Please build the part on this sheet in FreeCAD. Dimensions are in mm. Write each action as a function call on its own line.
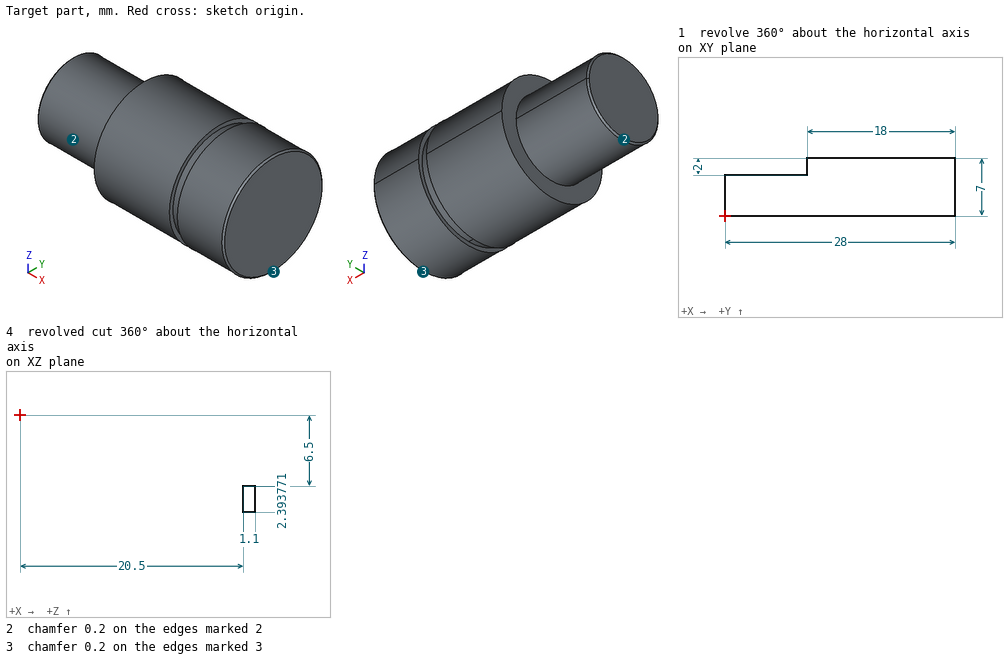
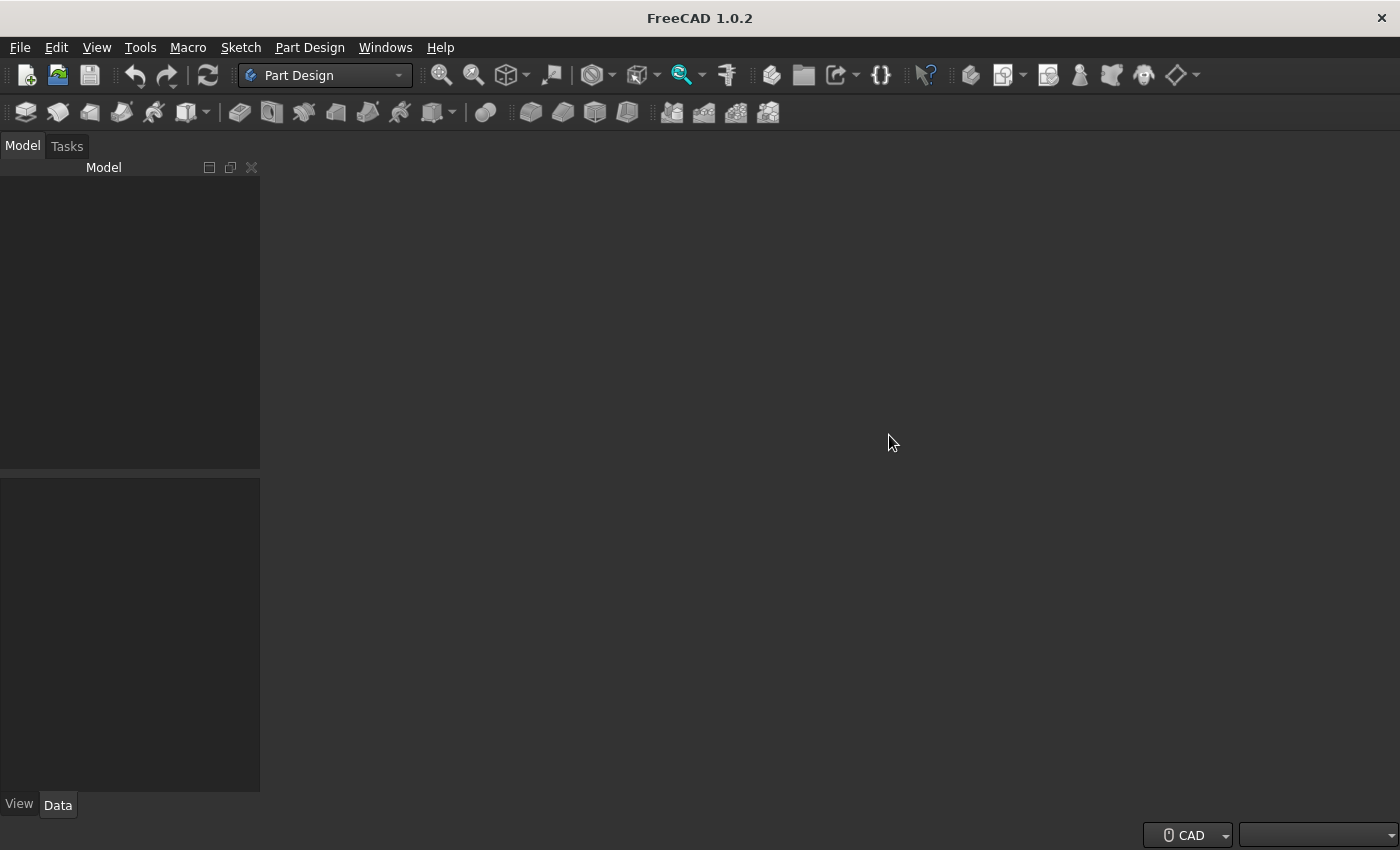
key(ctrl+n)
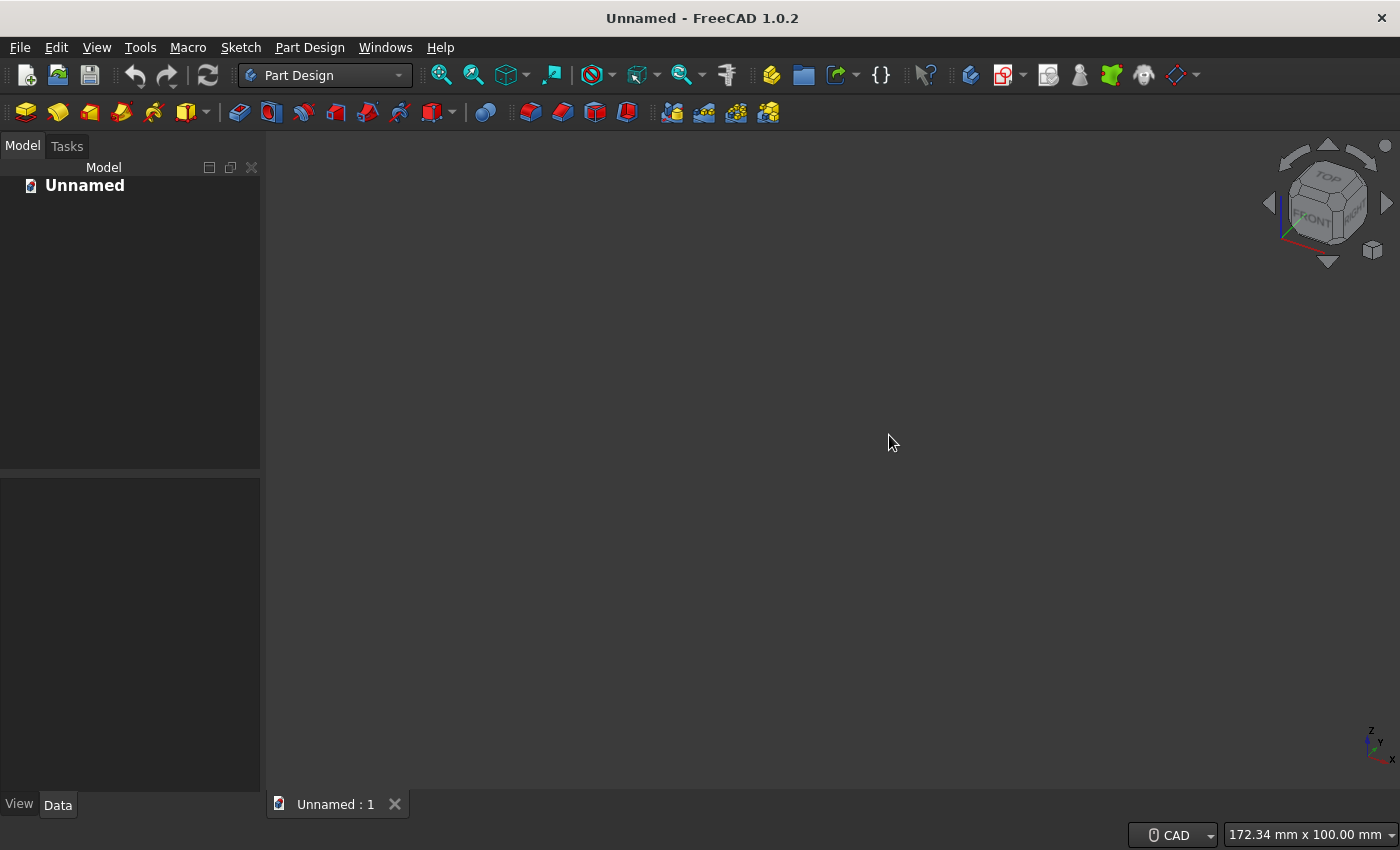
click(1004, 76)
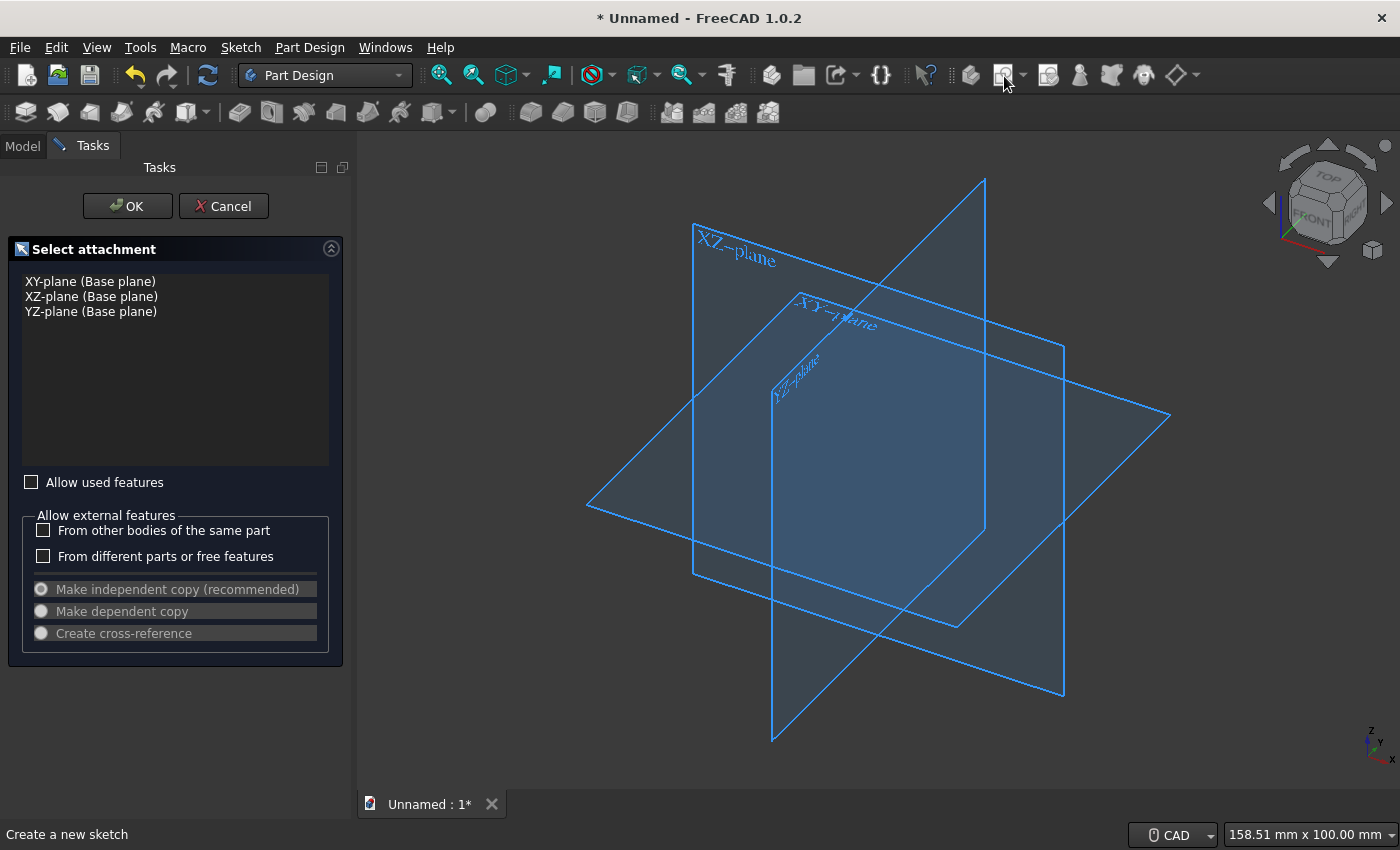
click(82, 282)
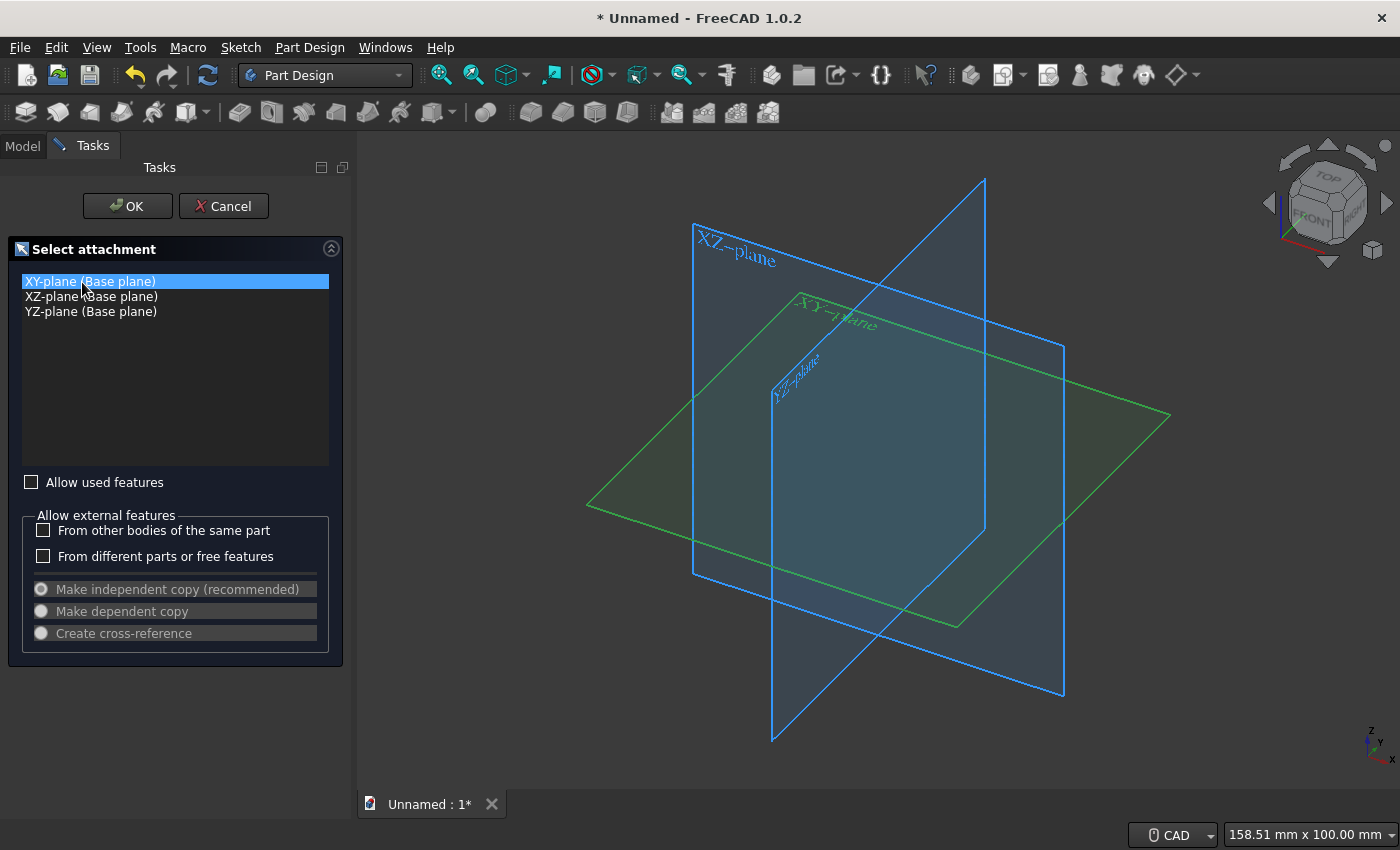
click(128, 206)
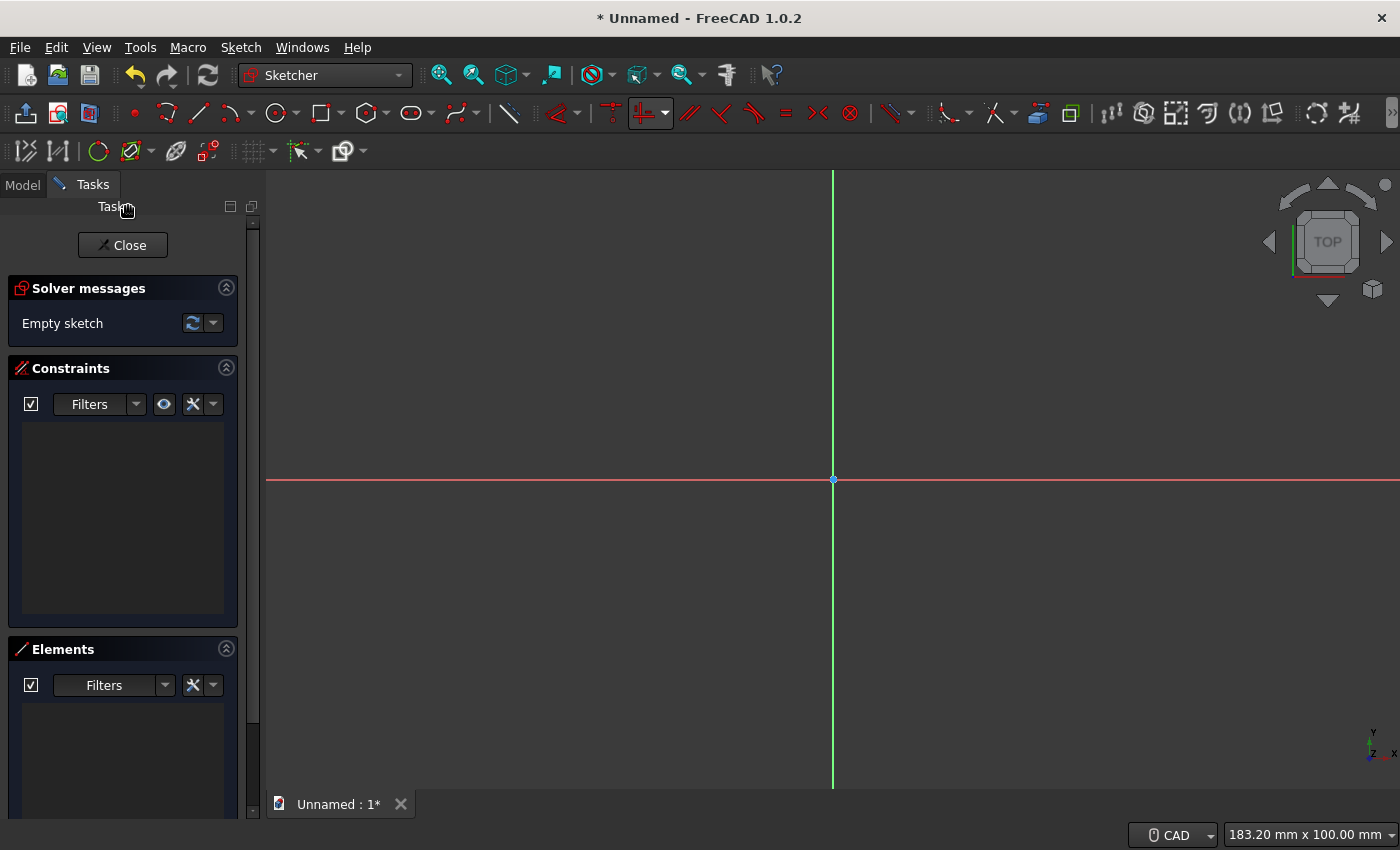
scroll(970, 451, up, 7)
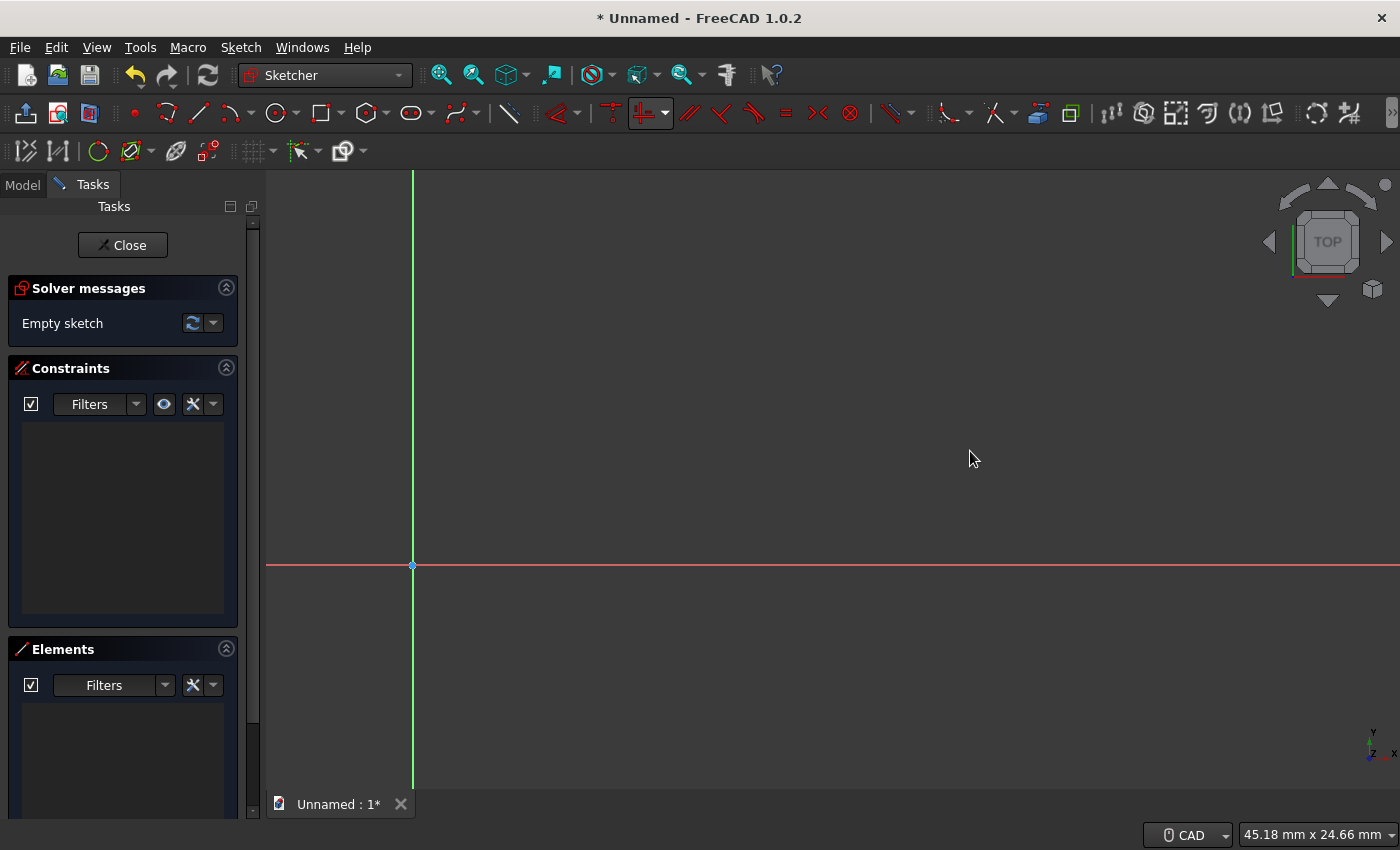
click(168, 114)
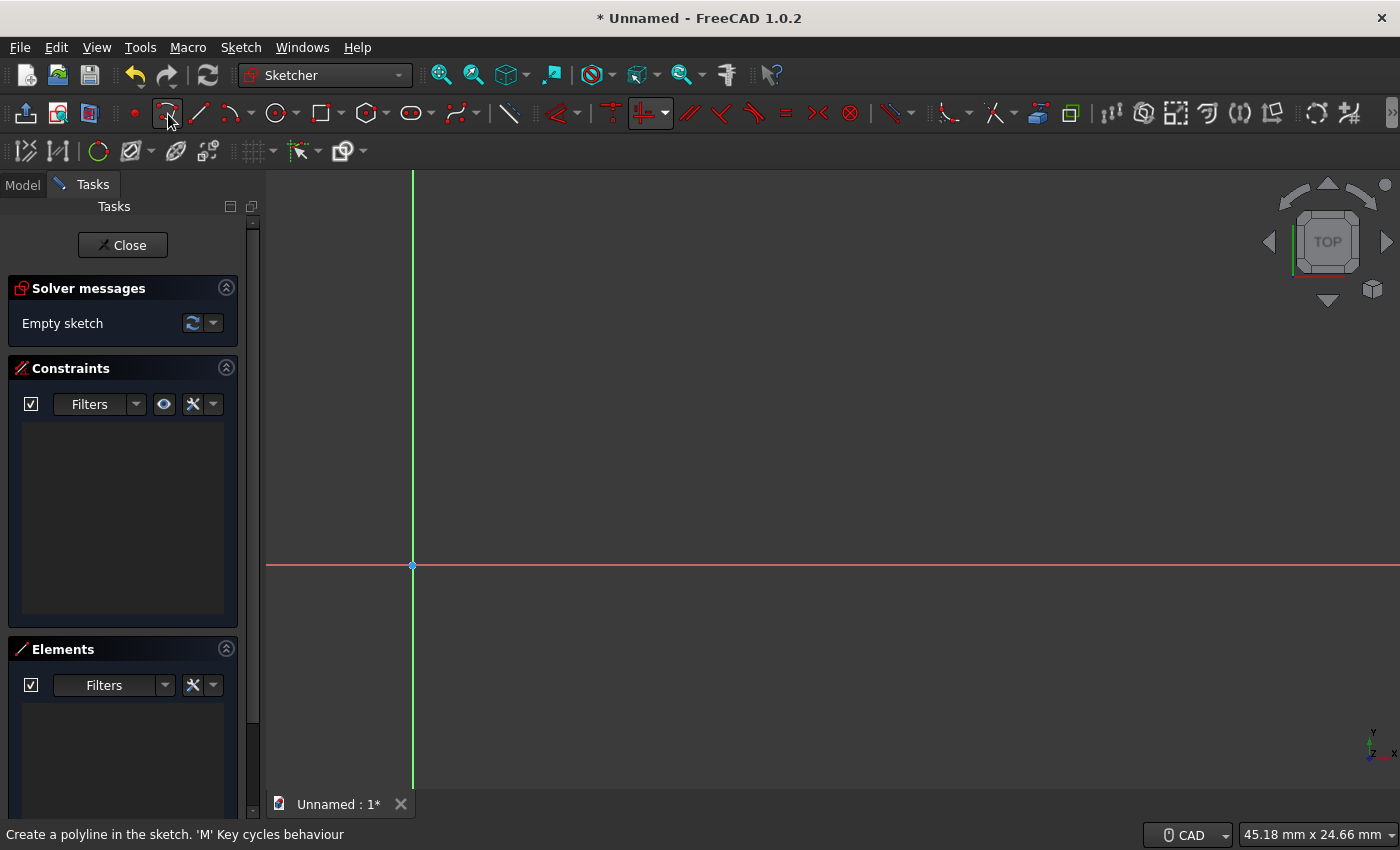
click(413, 565)
click(1115, 556)
click(1115, 389)
click(664, 389)
click(664, 440)
click(422, 440)
click(413, 565)
key(Escape)
key(Escape)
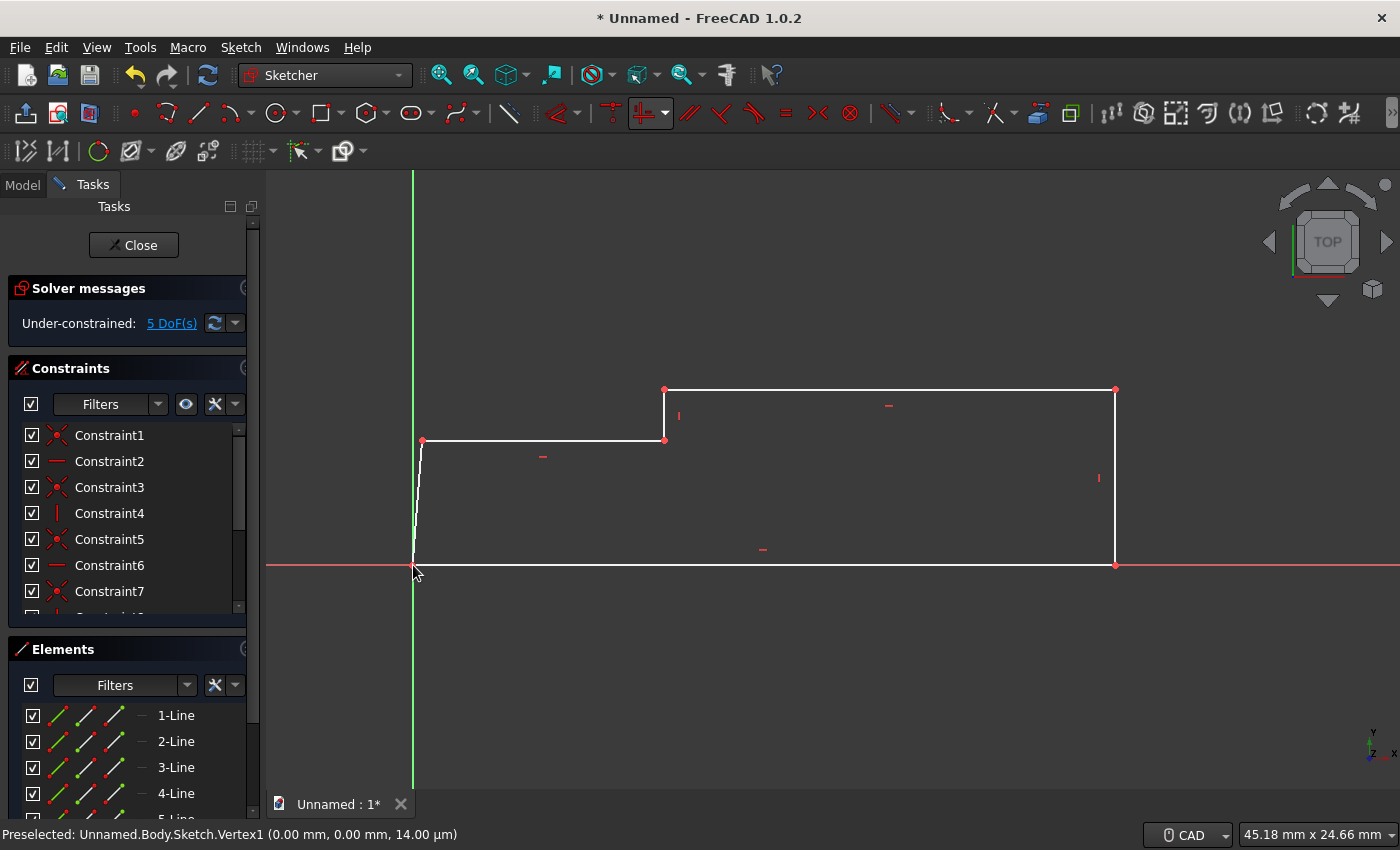
click(415, 528)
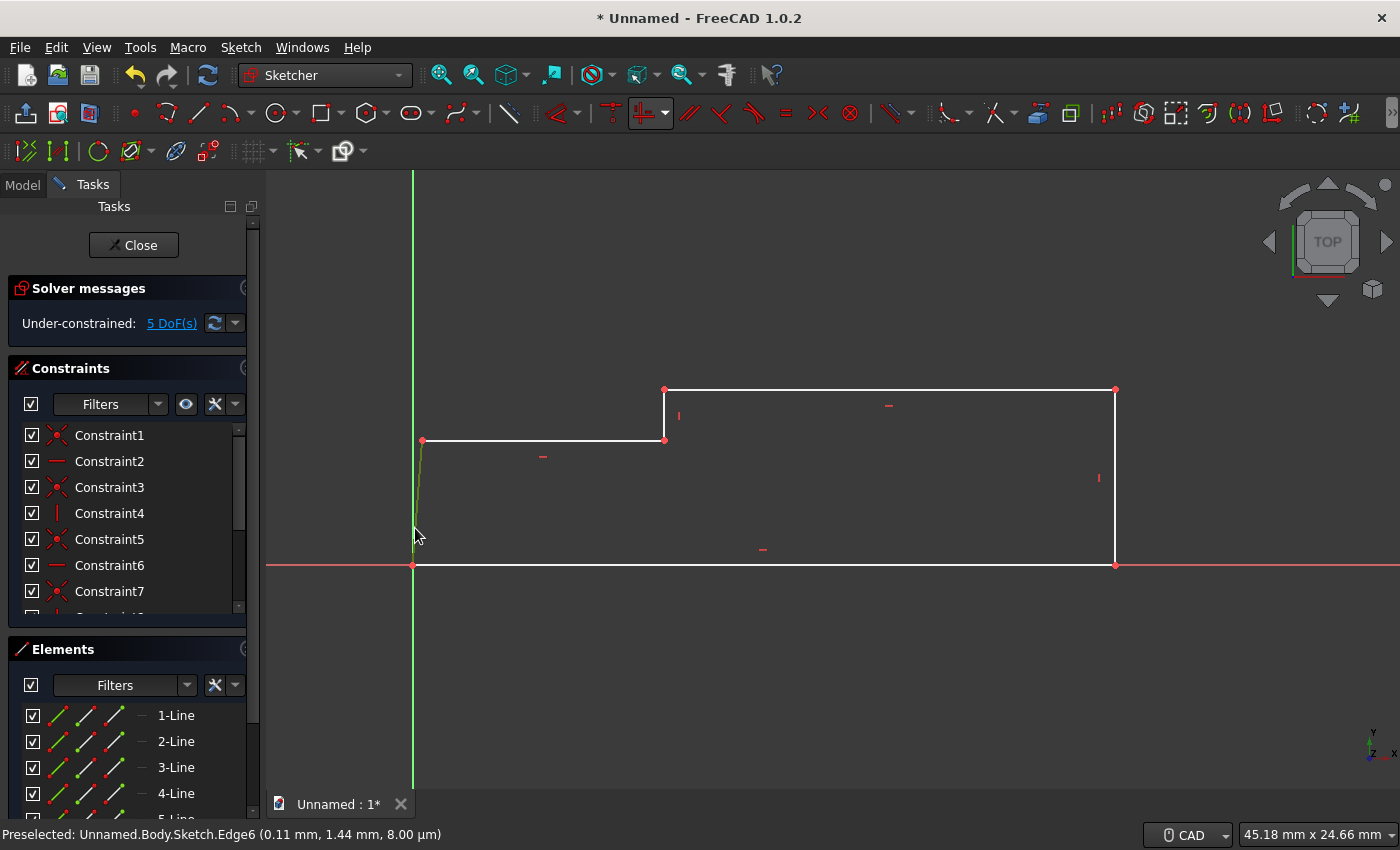
key(v)